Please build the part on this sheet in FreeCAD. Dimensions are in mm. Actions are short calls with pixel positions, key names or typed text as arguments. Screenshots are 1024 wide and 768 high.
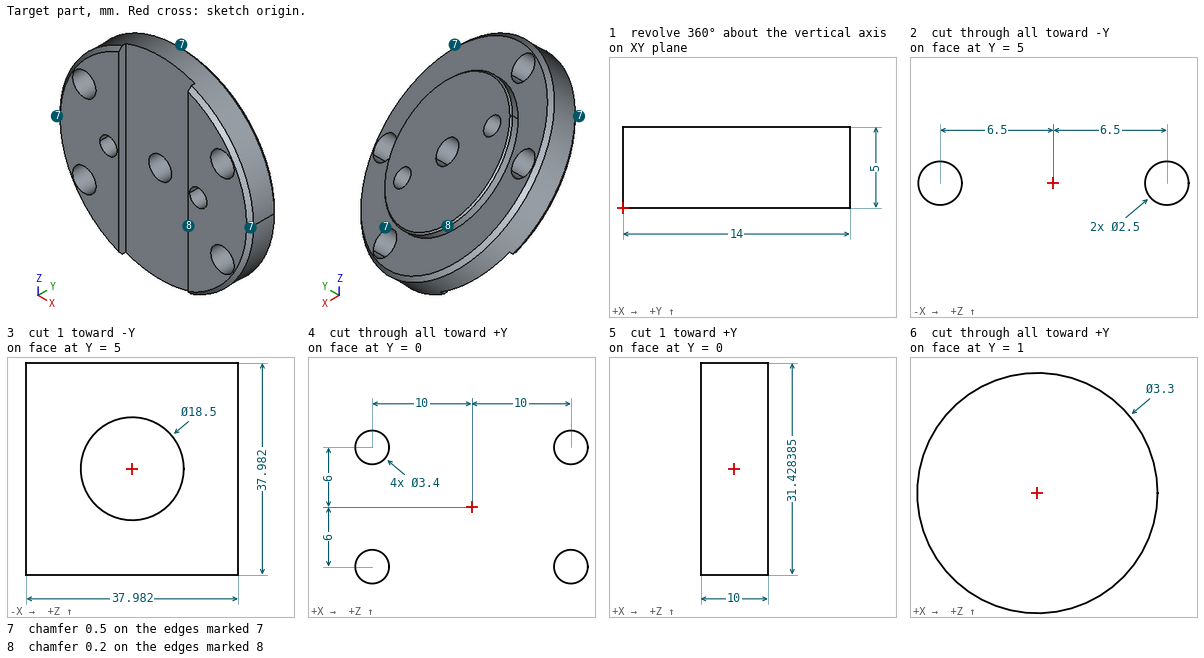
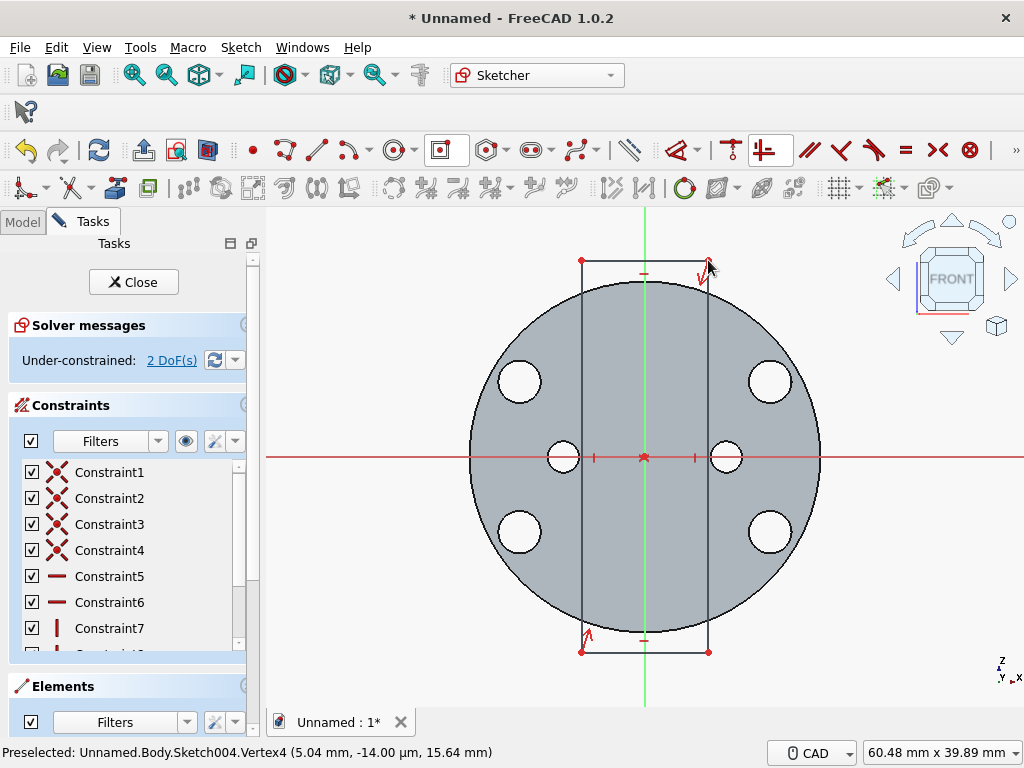
click(676, 150)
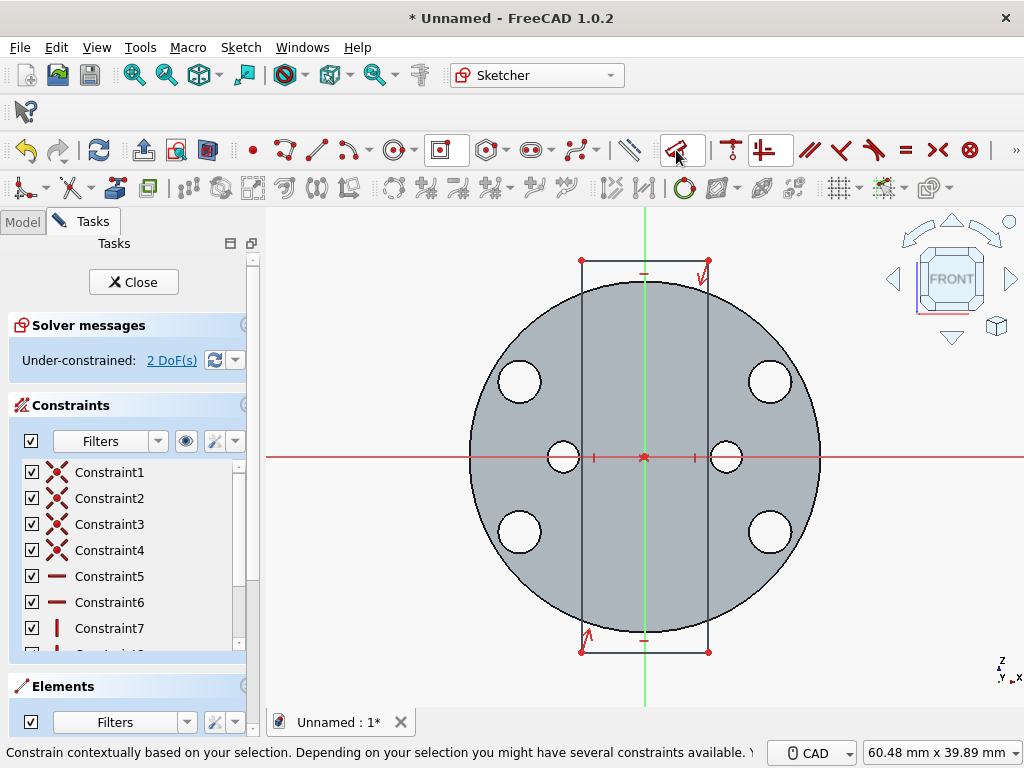
click(620, 653)
click(616, 619)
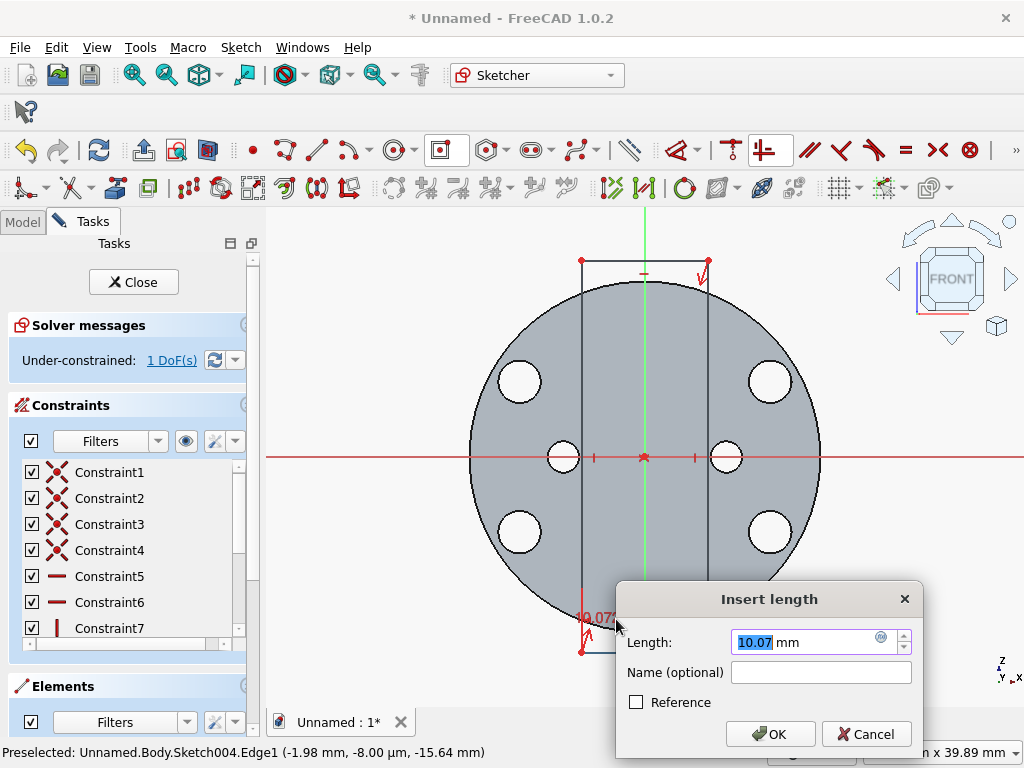
text(10)
key(Return)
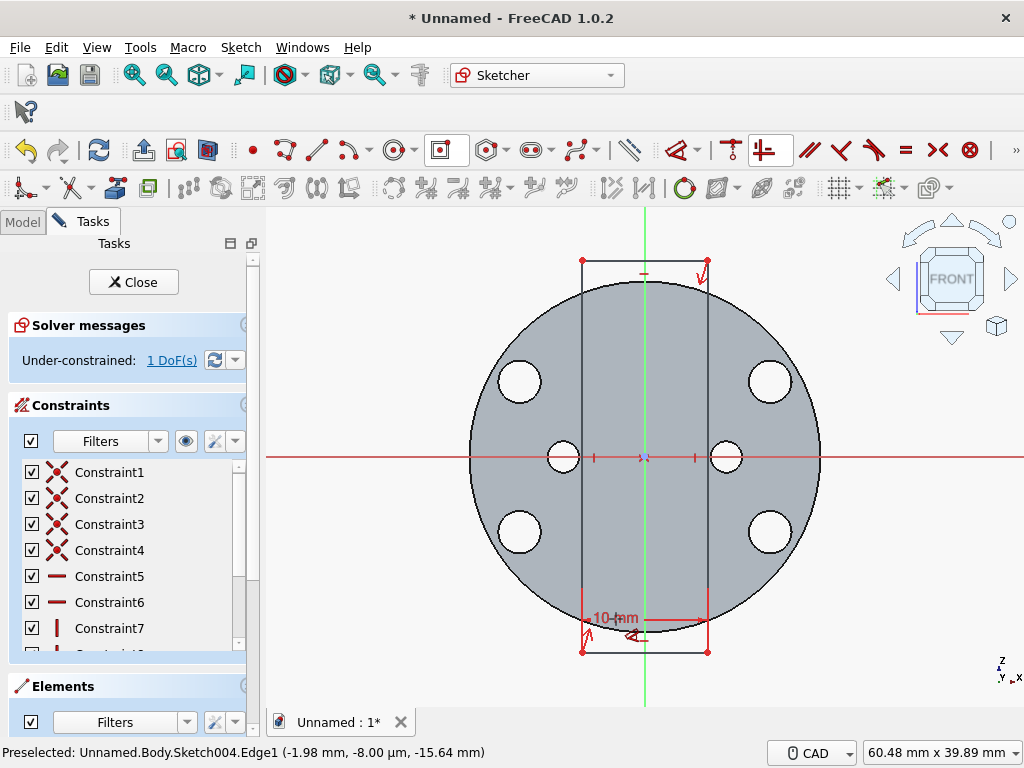
click(708, 535)
click(742, 367)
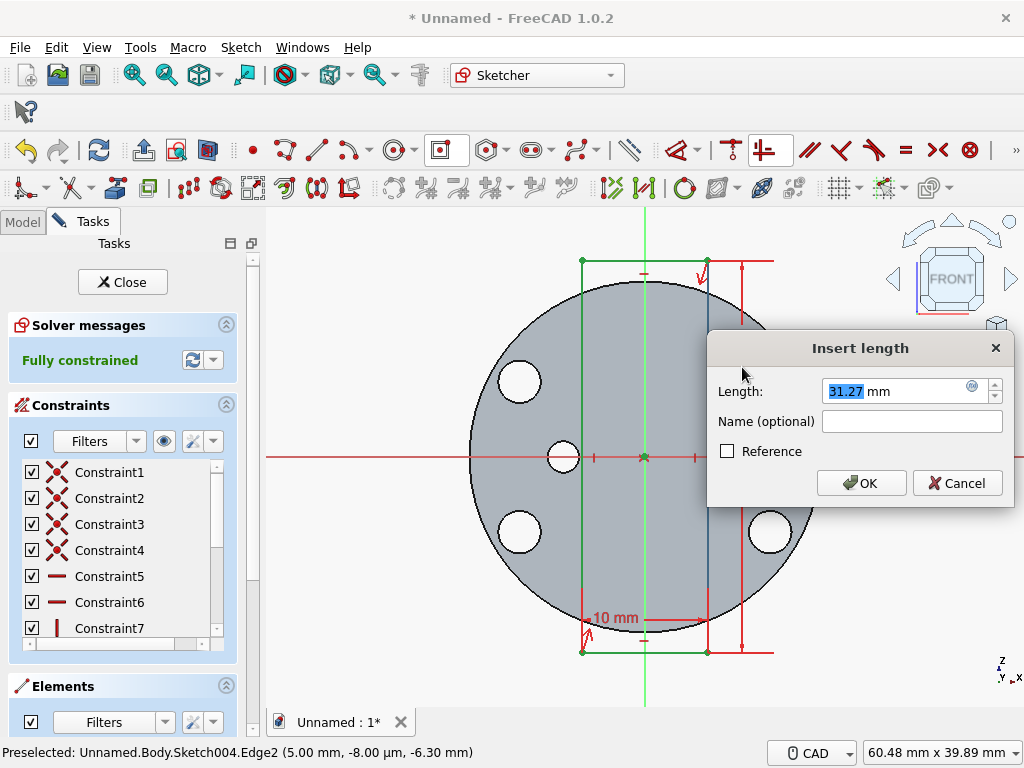
text(31.428385)
key(Return)
key(Escape)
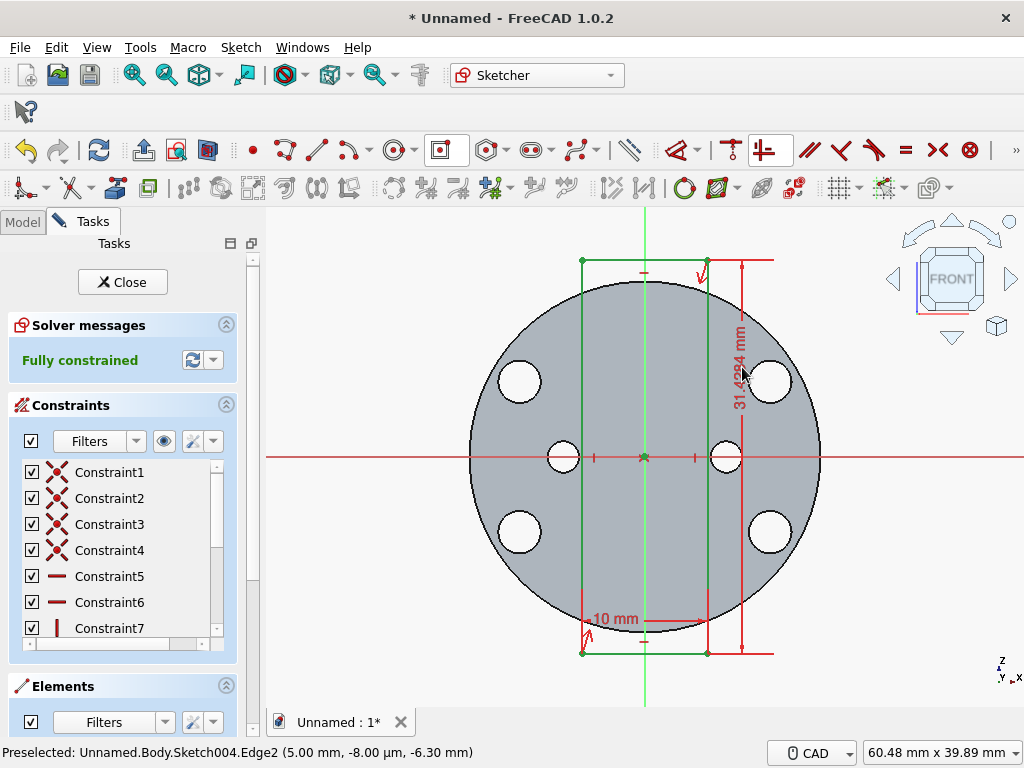
click(123, 282)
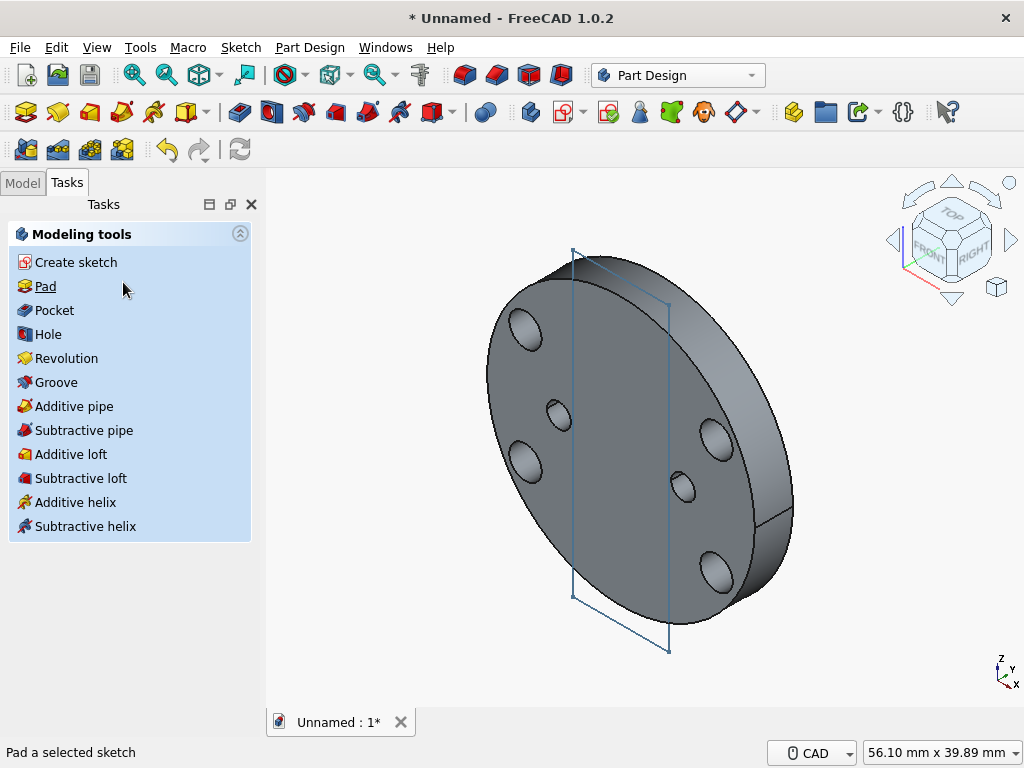
click(240, 112)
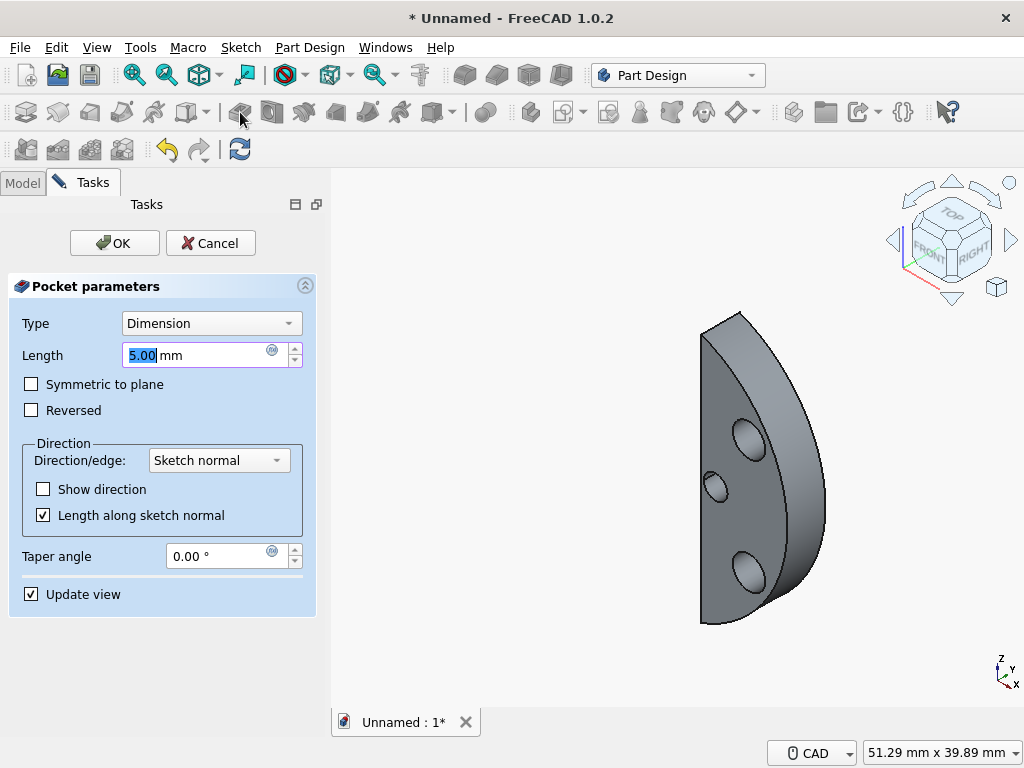
text(1)
key(Tab)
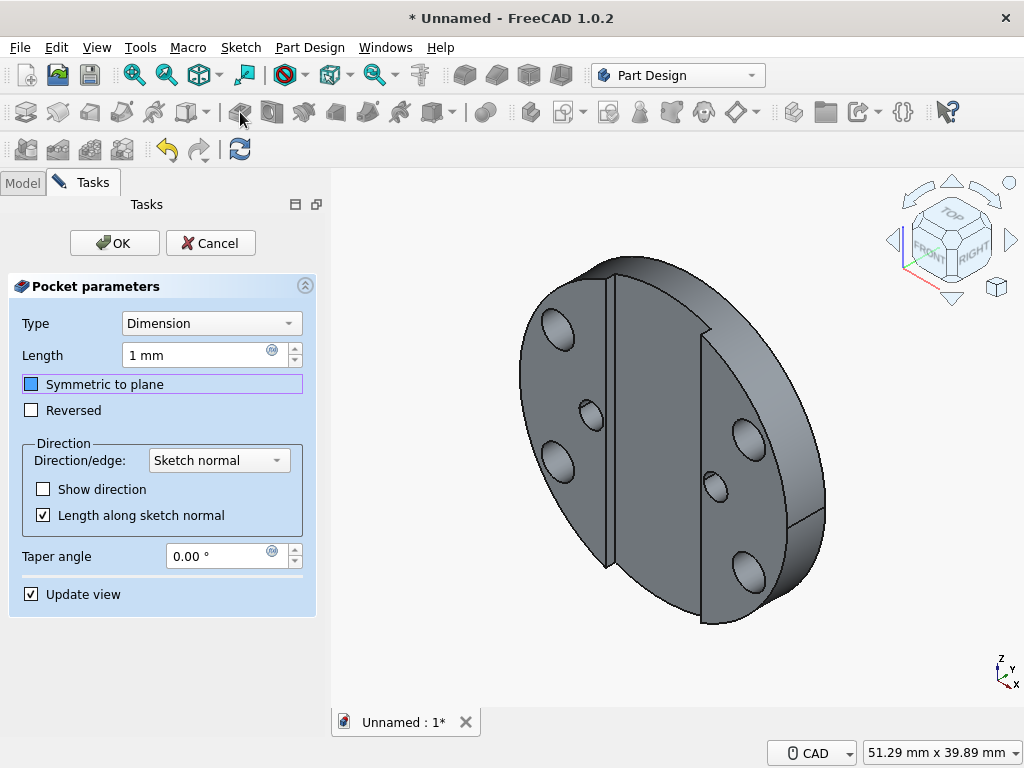
click(115, 243)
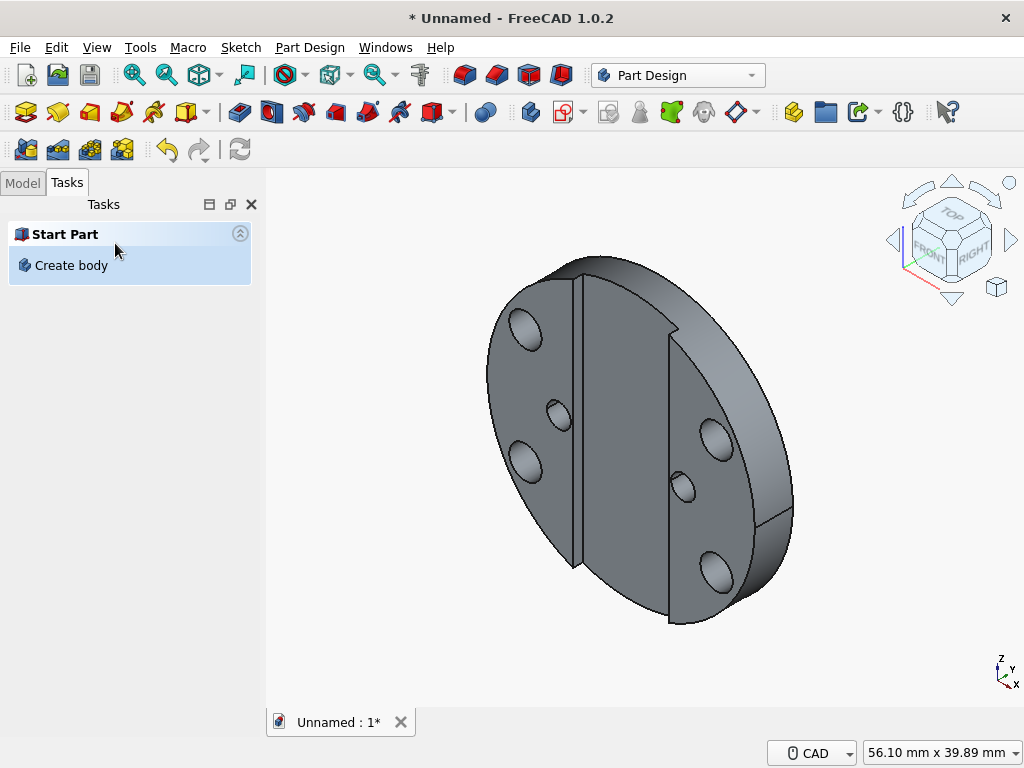
click(631, 356)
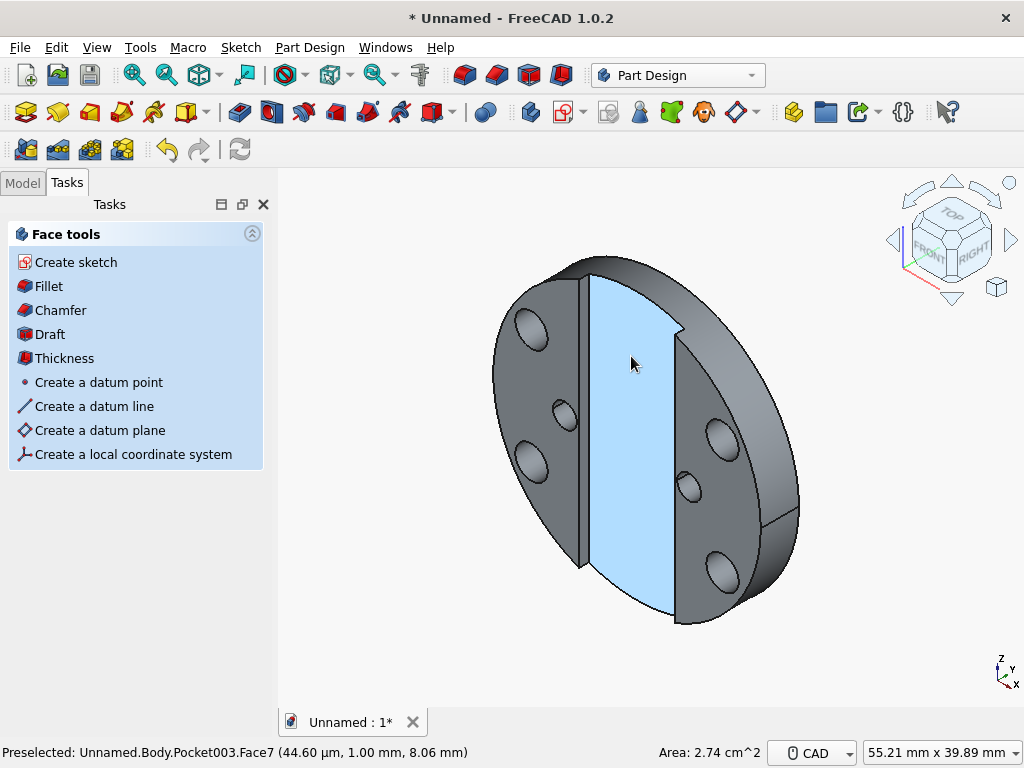
click(564, 112)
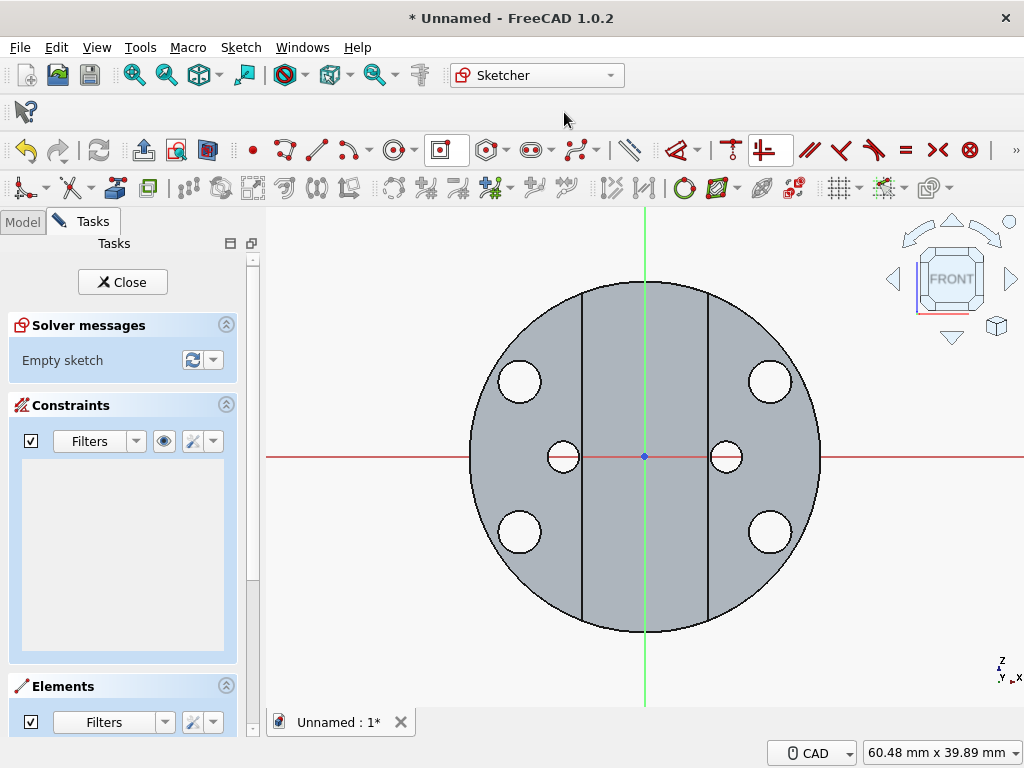
key(q)
key(s)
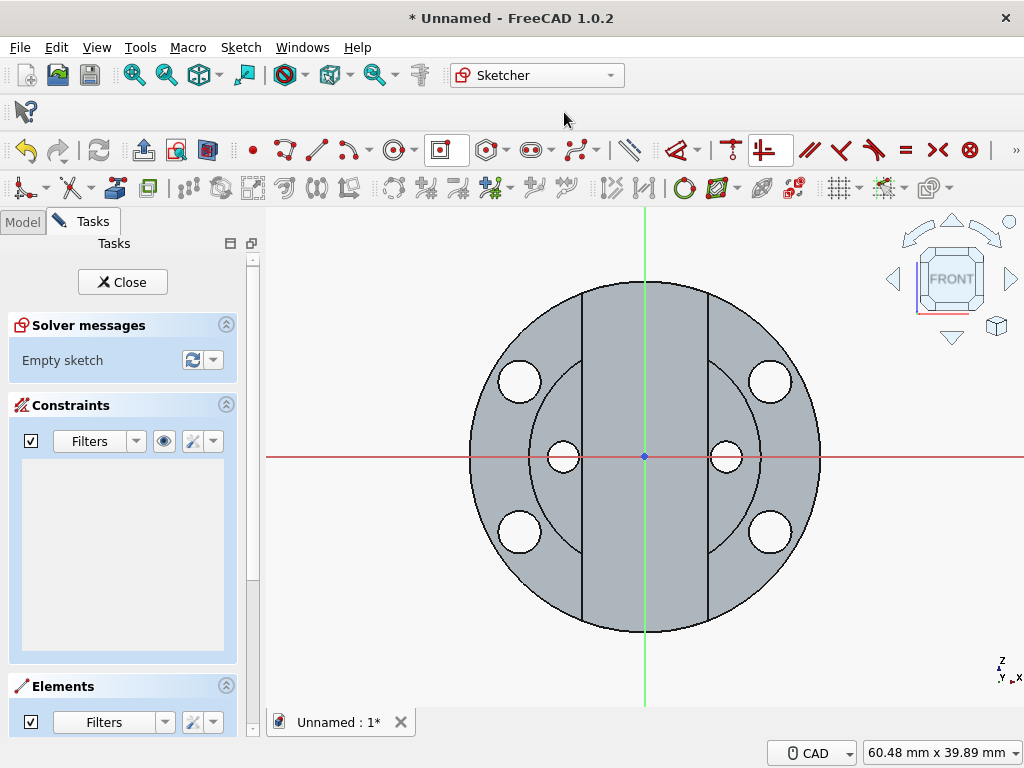
scroll(656, 457, up, 10)